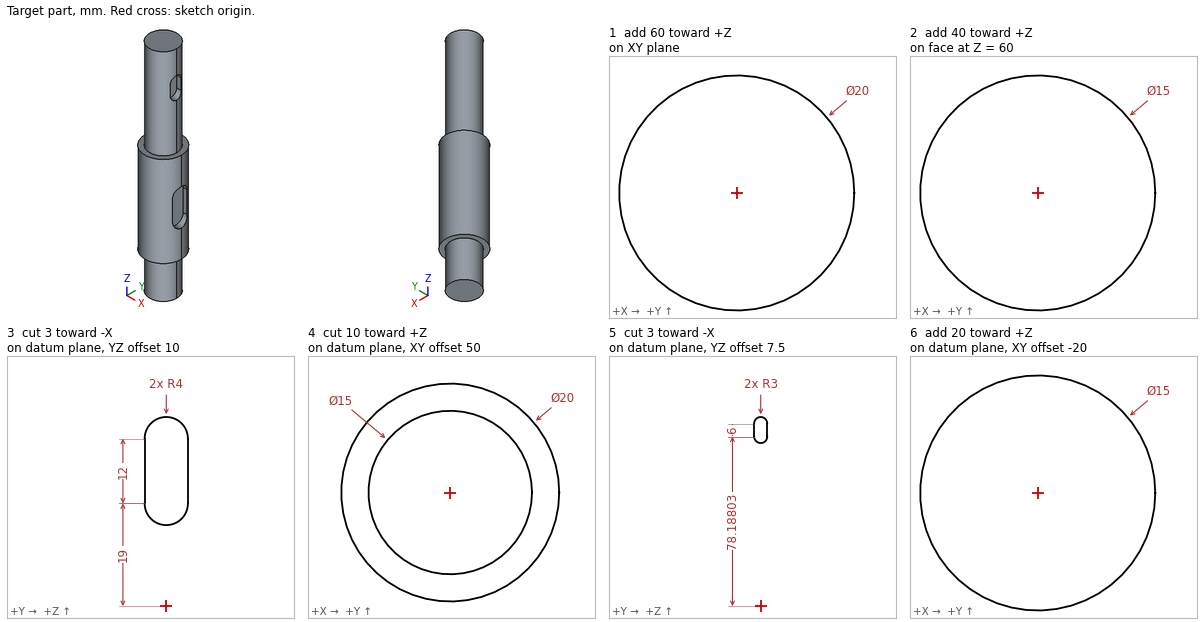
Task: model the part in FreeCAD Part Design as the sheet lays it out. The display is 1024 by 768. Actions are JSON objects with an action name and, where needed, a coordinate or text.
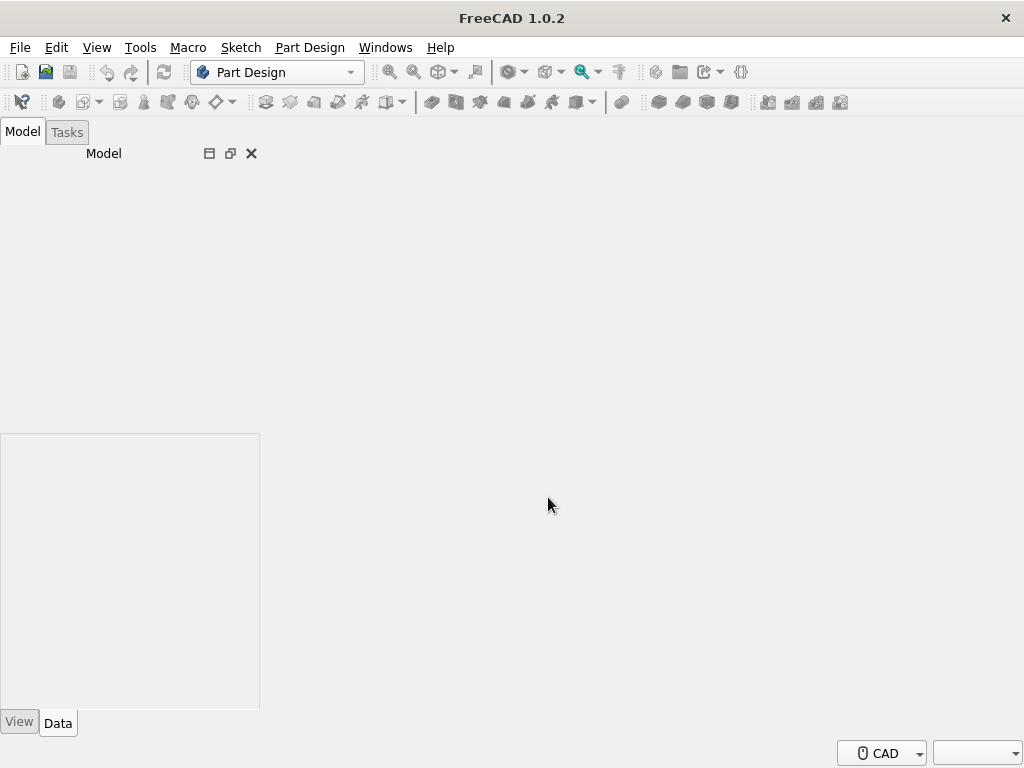
{"action": "left_click", "coordinate": [22, 72]}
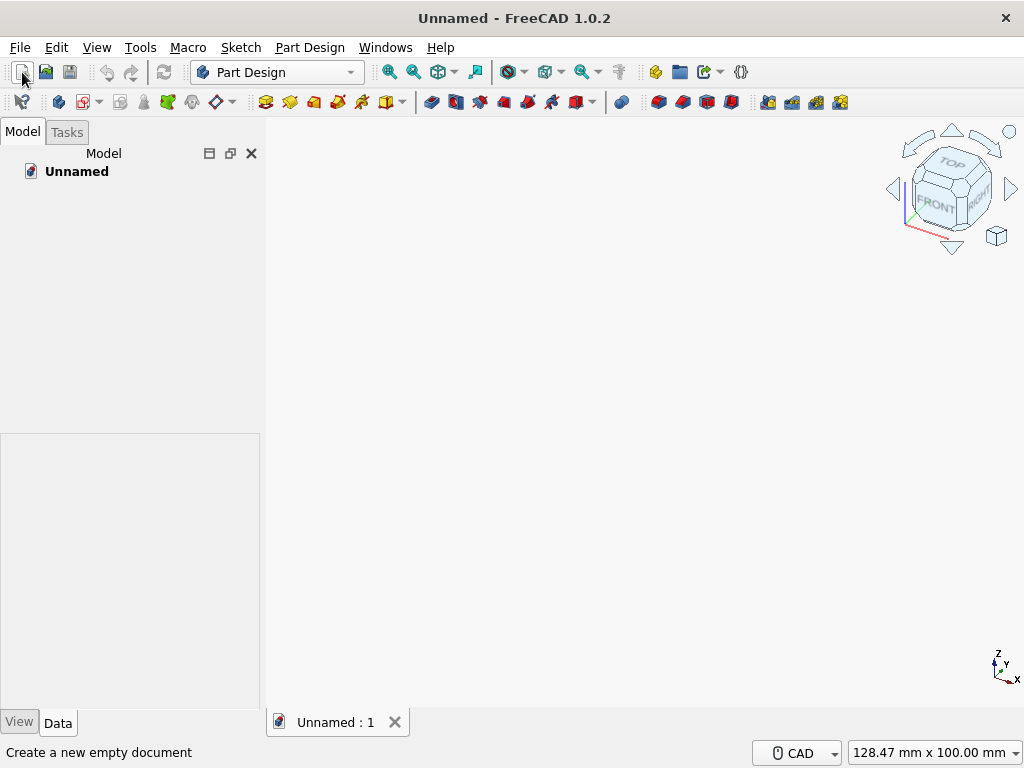
{"action": "left_click", "coordinate": [84, 102]}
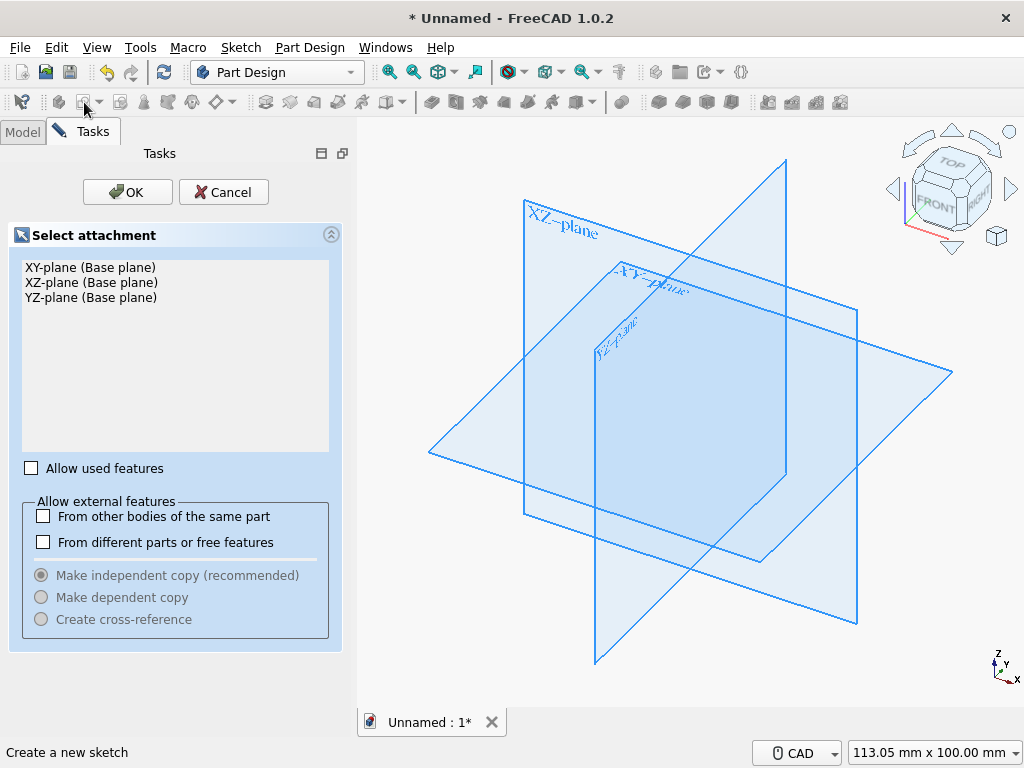
{"action": "left_click", "coordinate": [82, 268]}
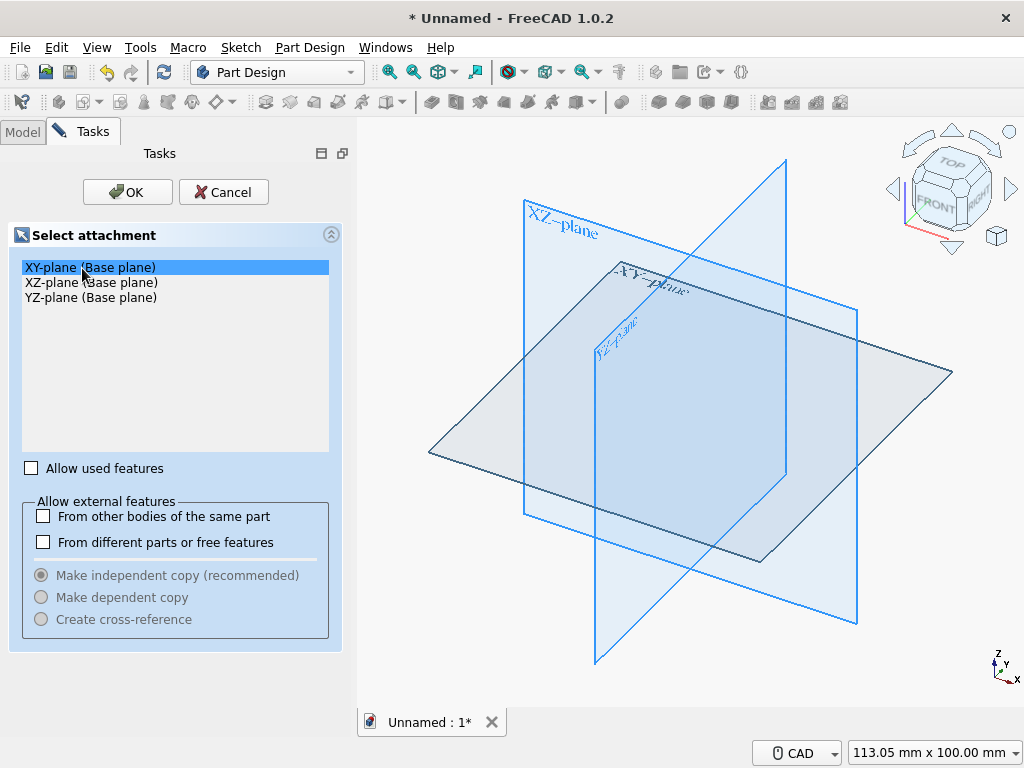
{"action": "left_click", "coordinate": [128, 192]}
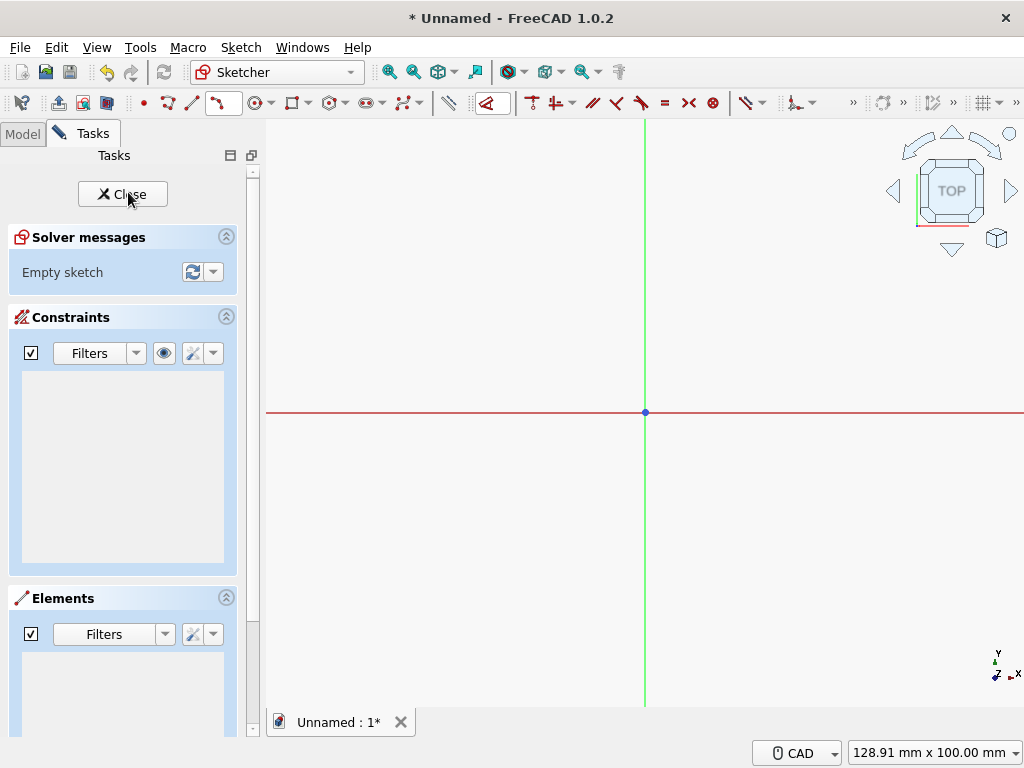
{"action": "scroll", "coordinate": [675, 413], "scroll_direction": "up", "scroll_amount": 6}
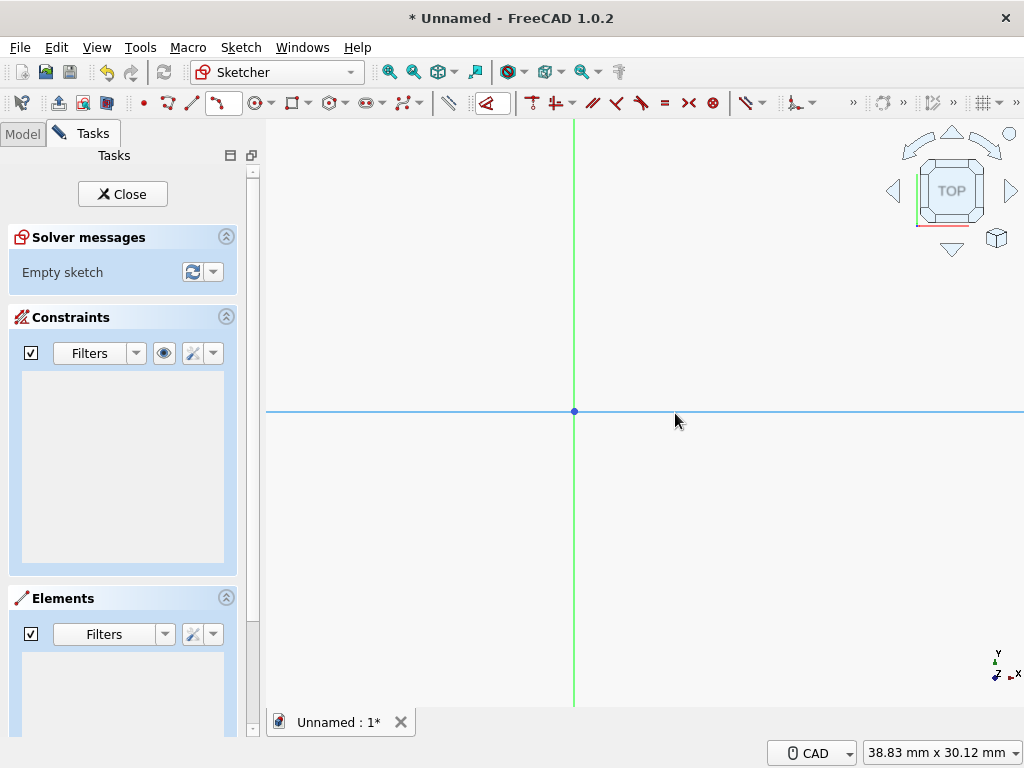
{"action": "left_click", "coordinate": [256, 104]}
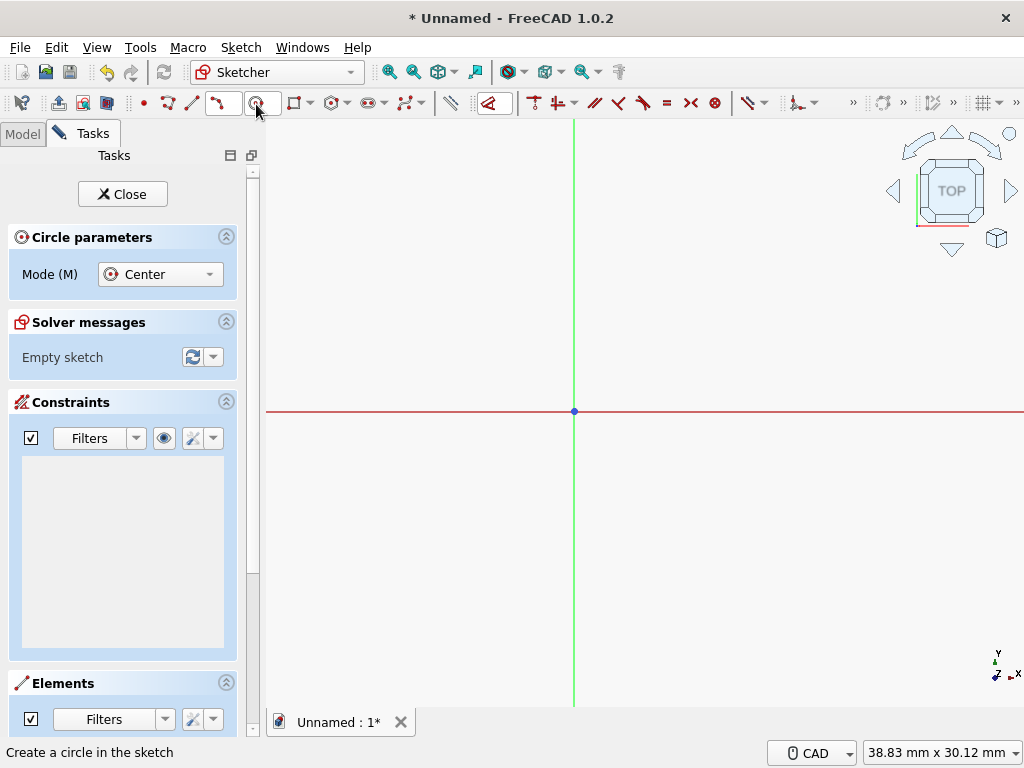
{"action": "left_click", "coordinate": [574, 412]}
{"action": "mouse_move", "coordinate": [712, 274]}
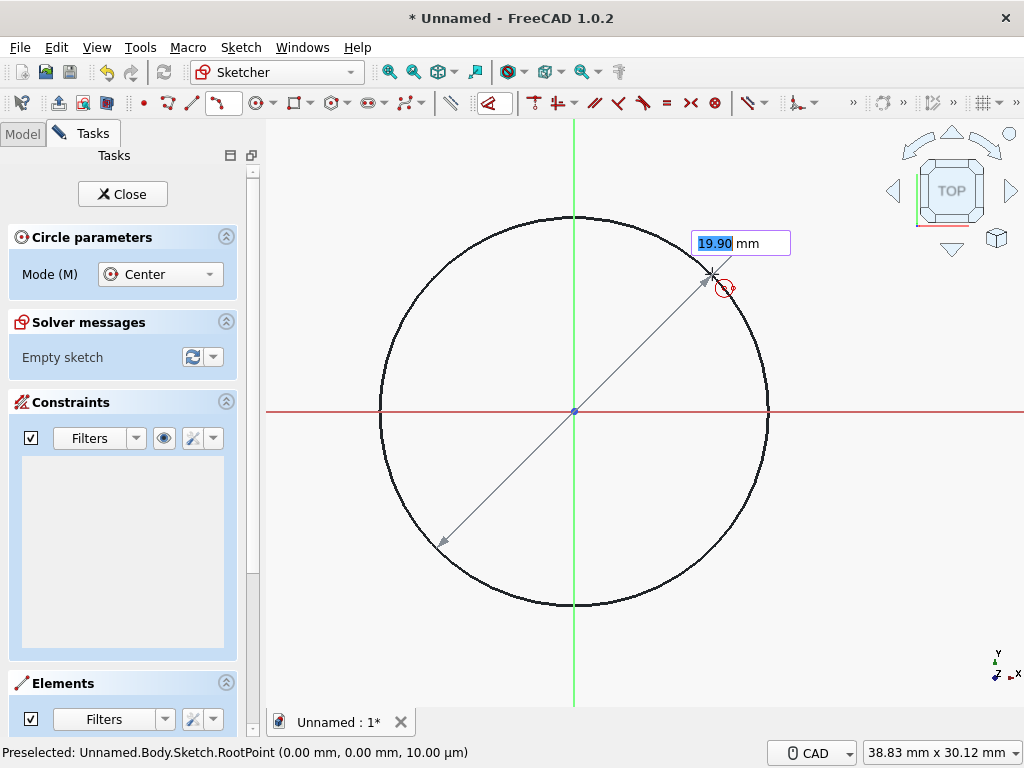
{"action": "type", "text": "20"}
{"action": "key", "text": "Return"}
{"action": "key", "text": "Escape"}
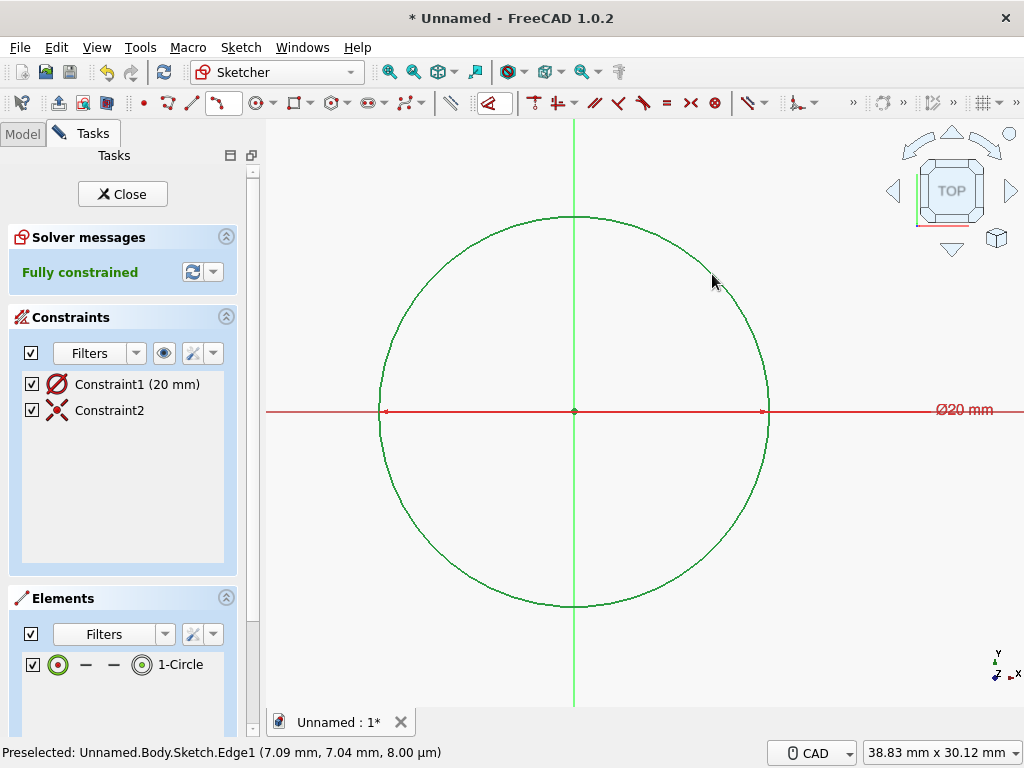
{"action": "left_click", "coordinate": [123, 194]}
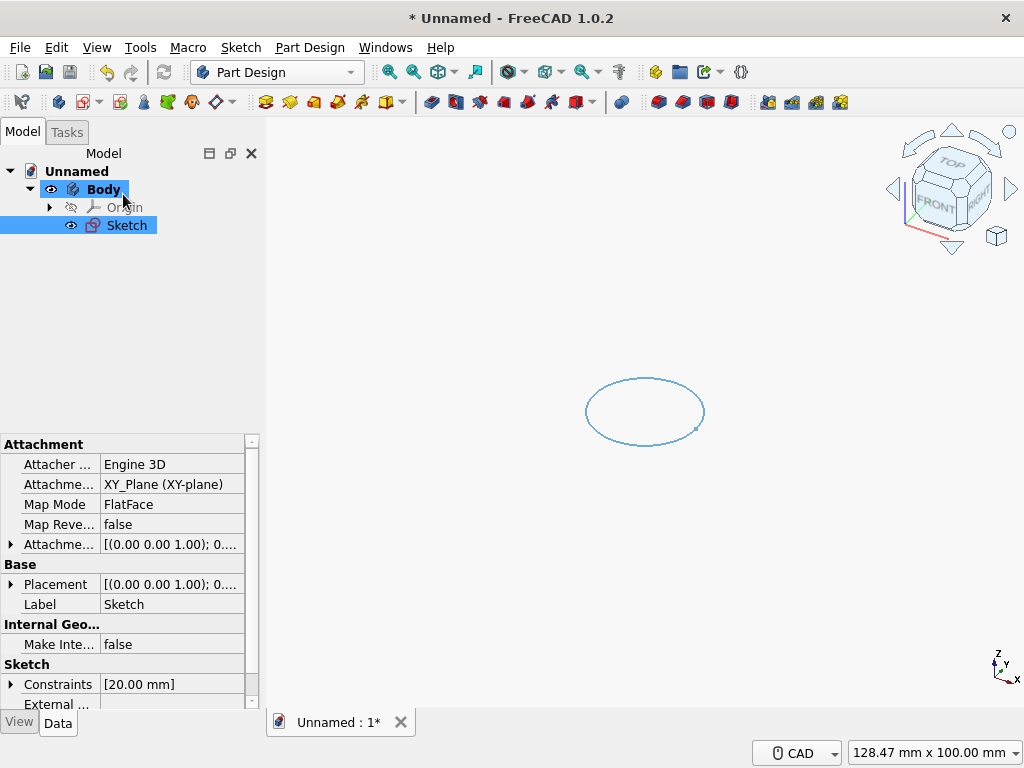
{"action": "left_click", "coordinate": [266, 102]}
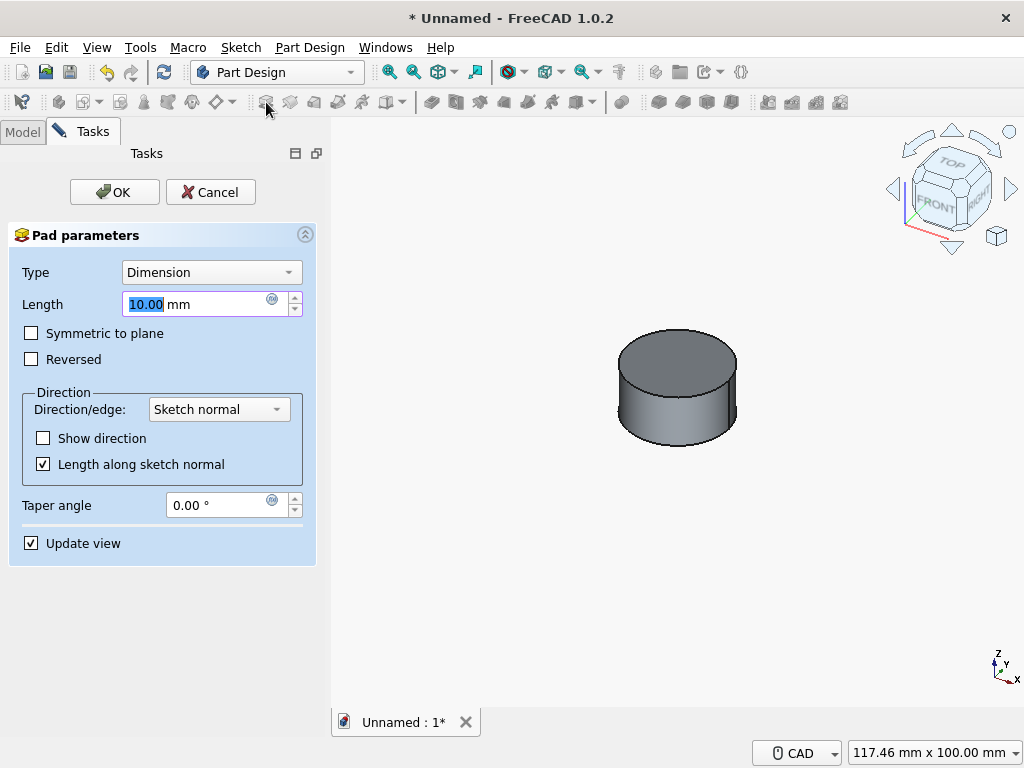
{"action": "type", "text": "60"}
{"action": "key", "text": "Tab"}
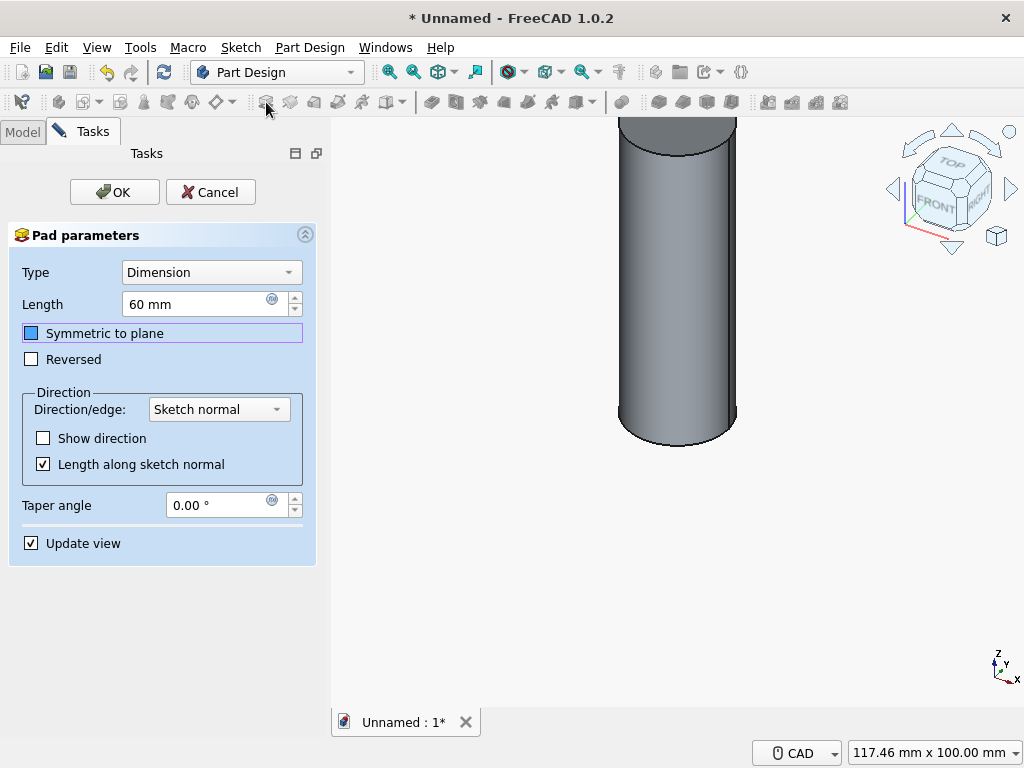
{"action": "left_click", "coordinate": [115, 192]}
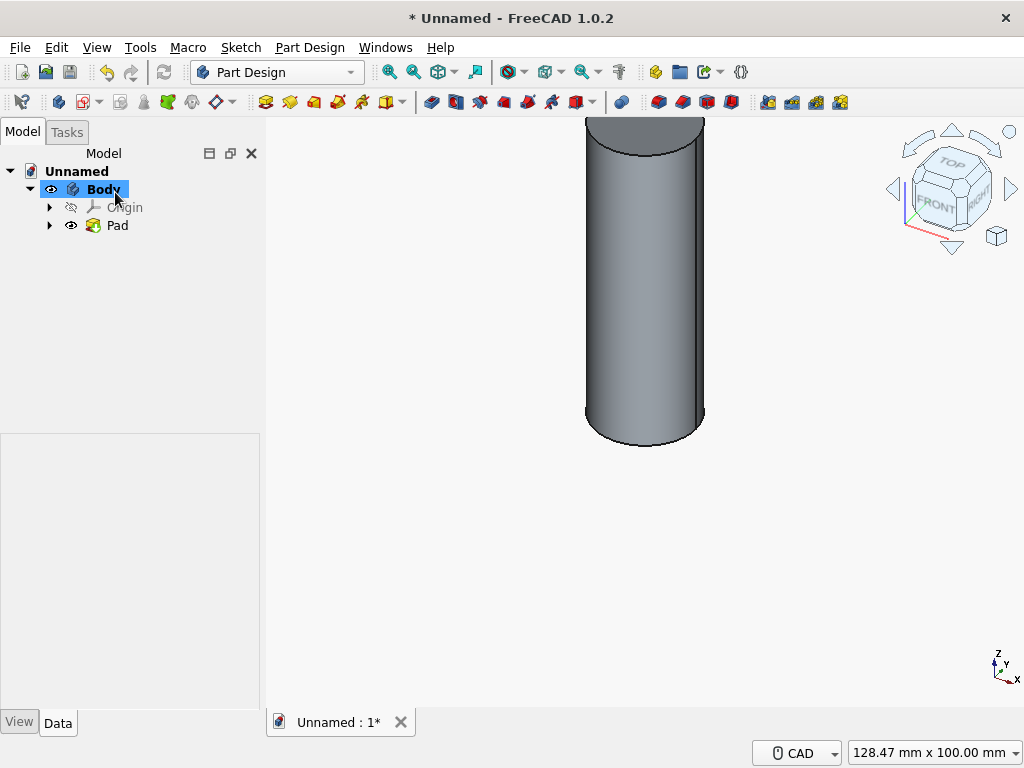
{"action": "left_click", "coordinate": [390, 72]}